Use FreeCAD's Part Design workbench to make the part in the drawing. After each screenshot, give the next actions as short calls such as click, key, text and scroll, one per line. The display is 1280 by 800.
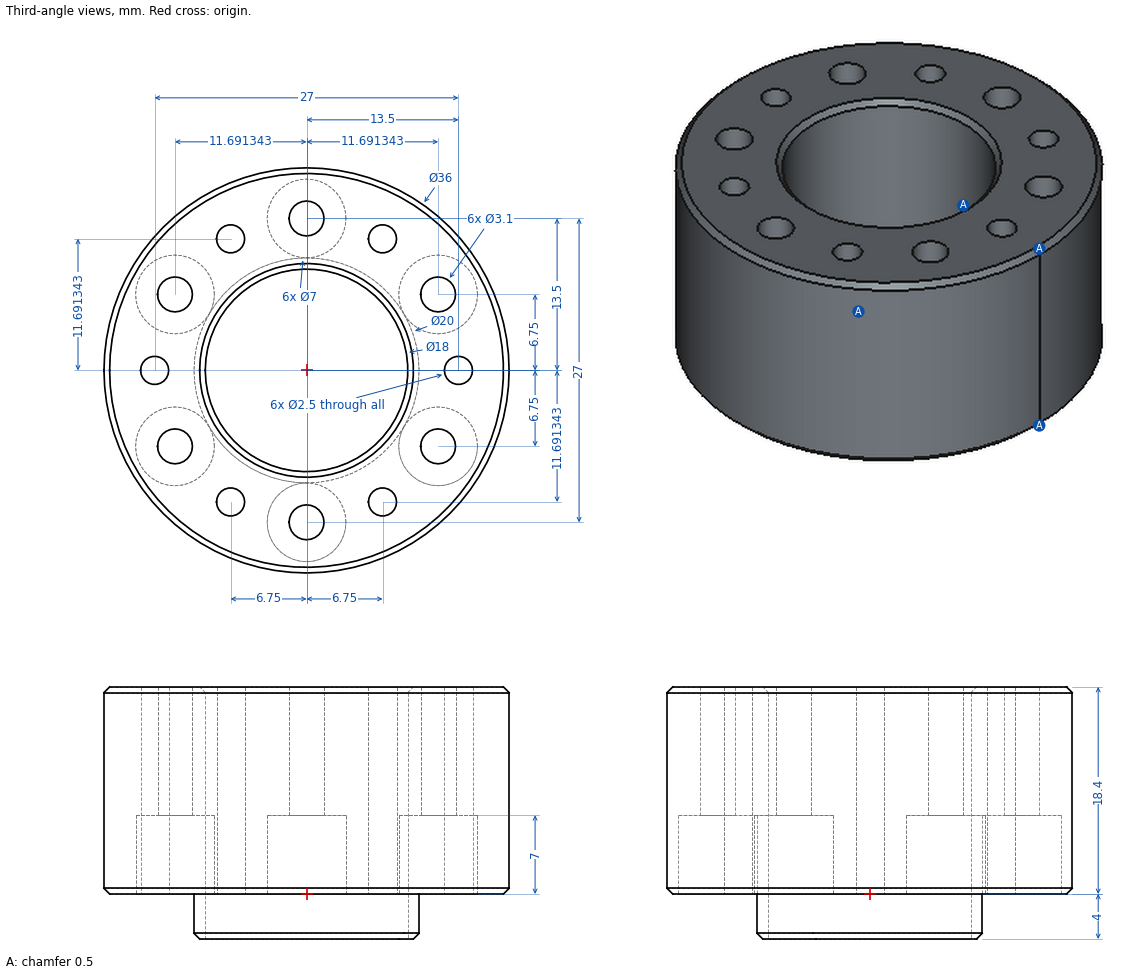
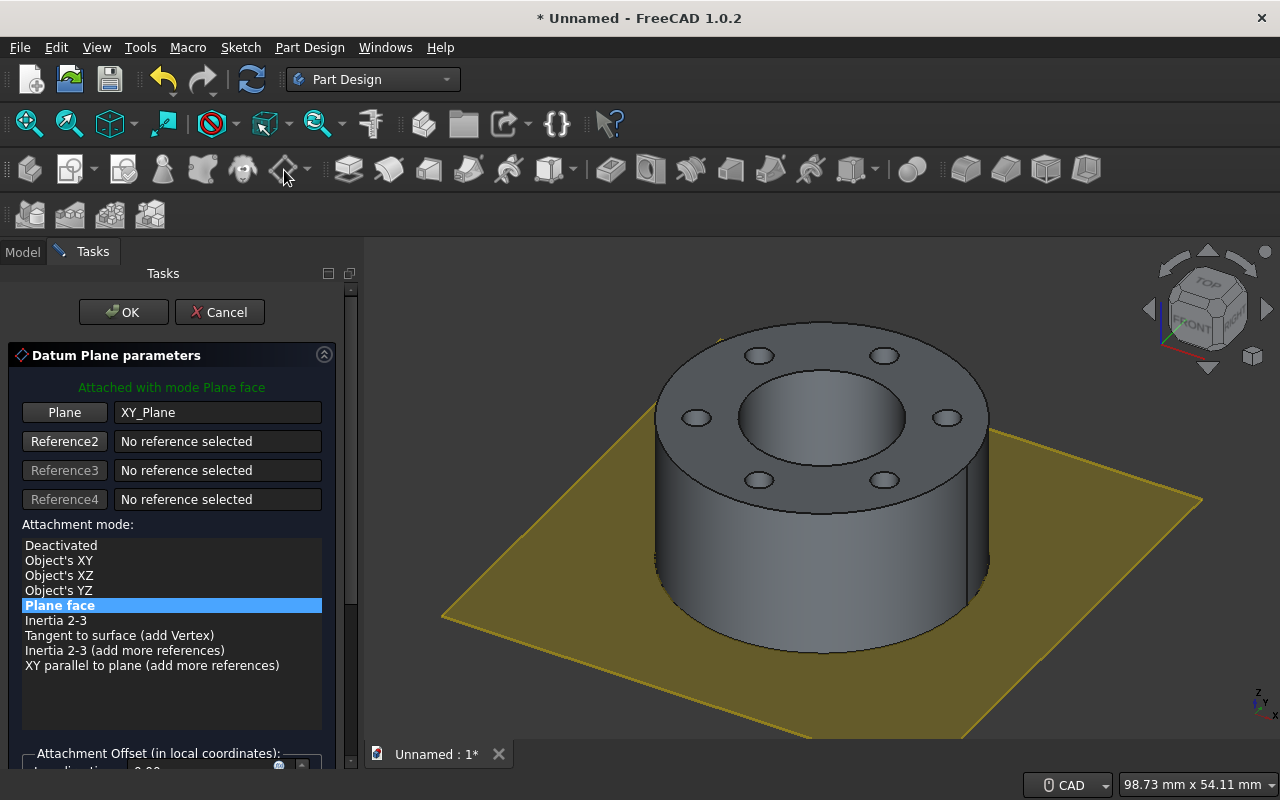
scroll(351, 526, down, 3)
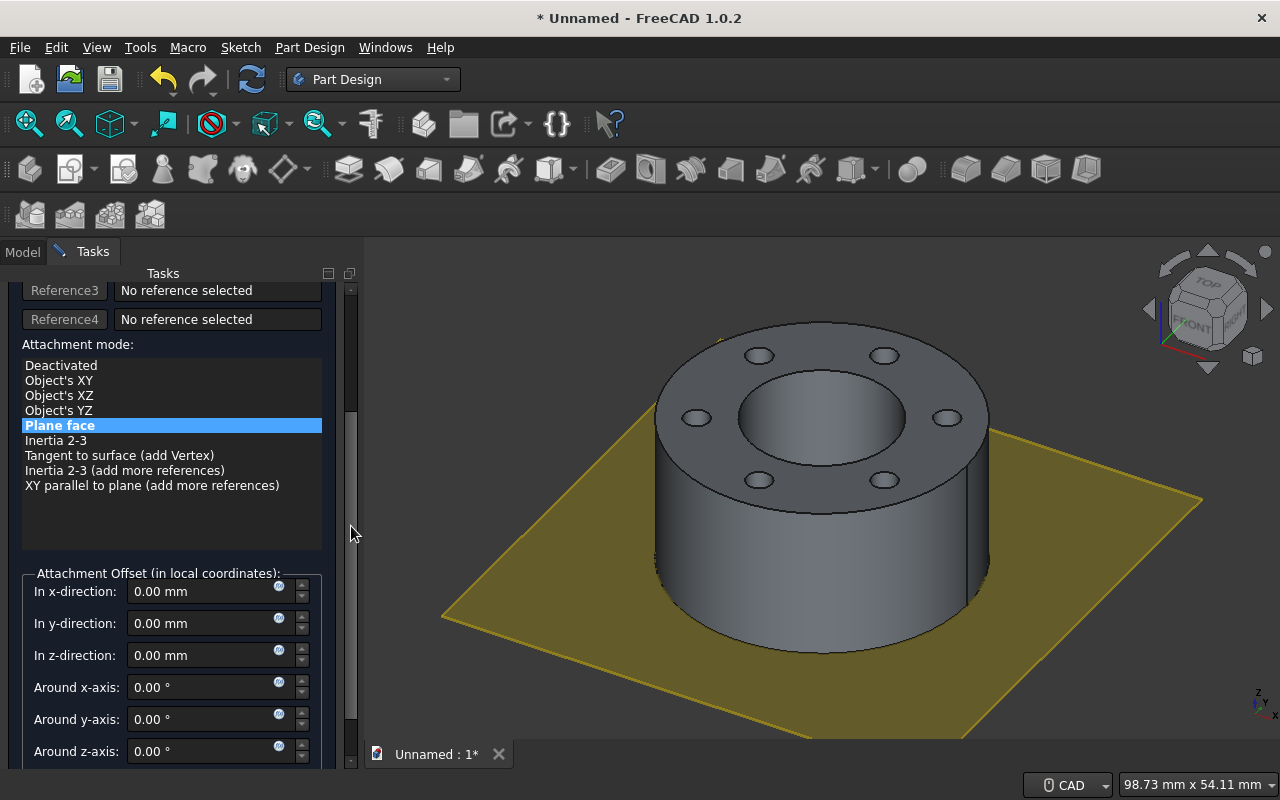
triple_click(210, 655)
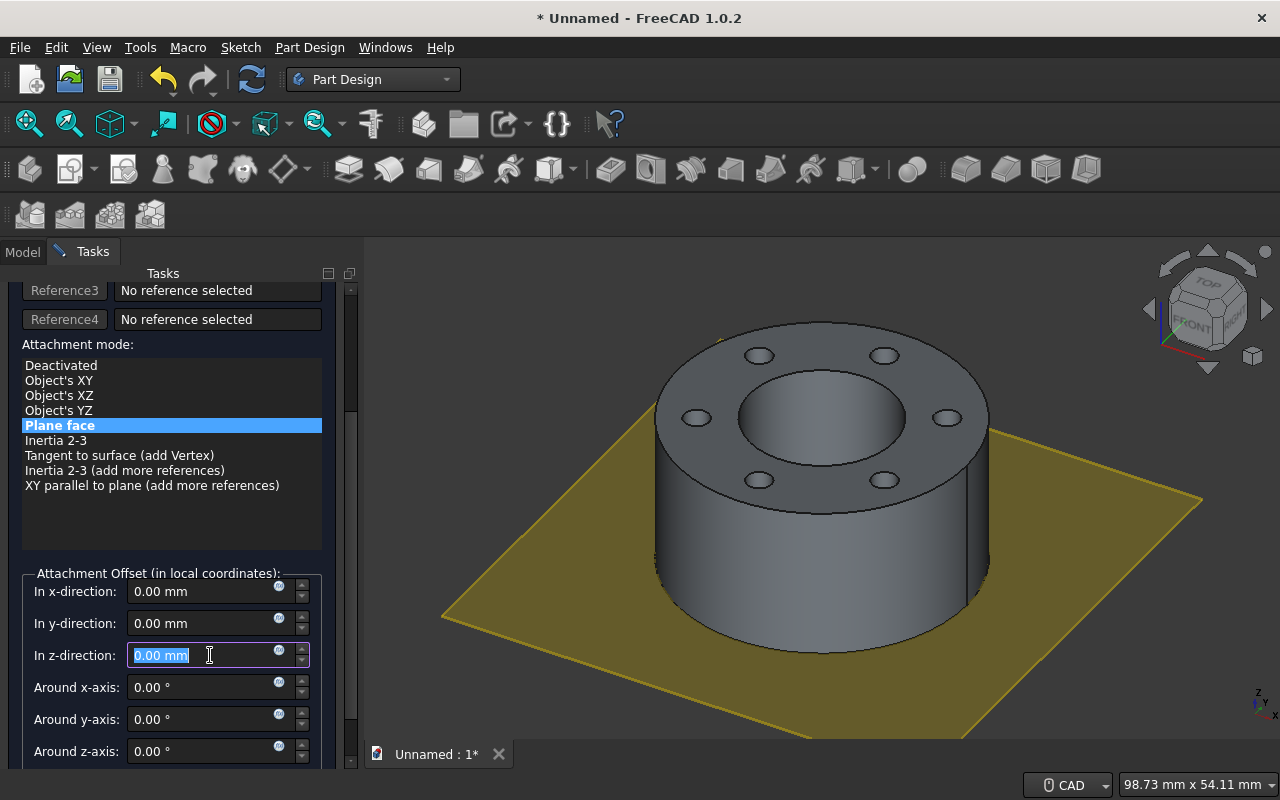
text(-4)
key(Tab)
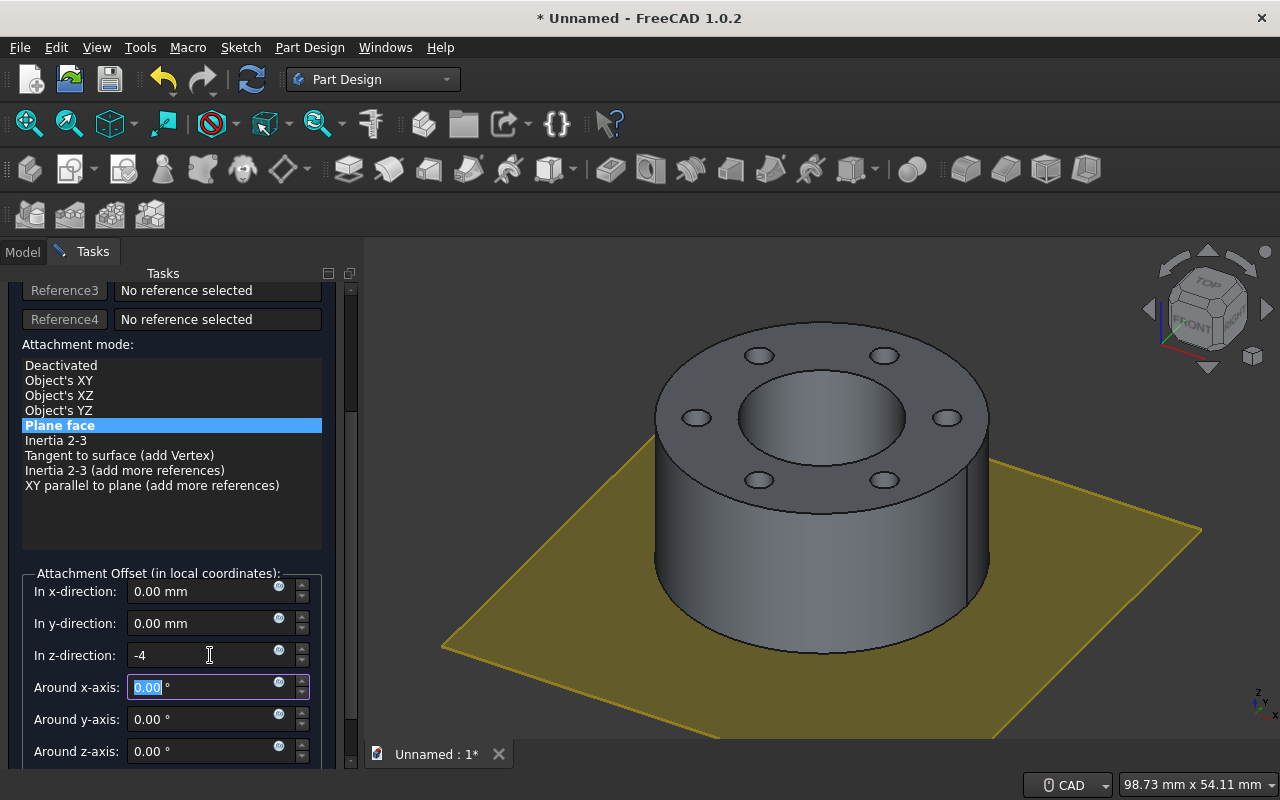
scroll(351, 526, up, 4)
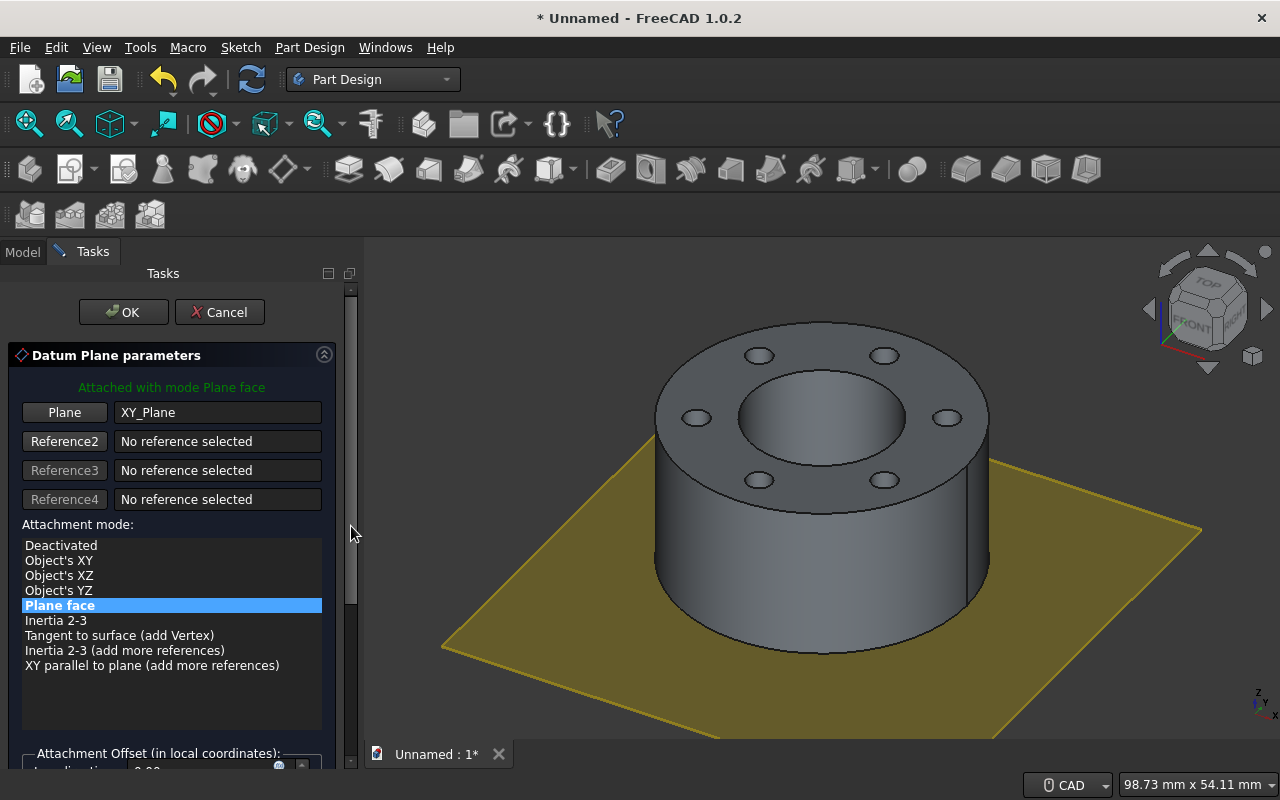
click(124, 312)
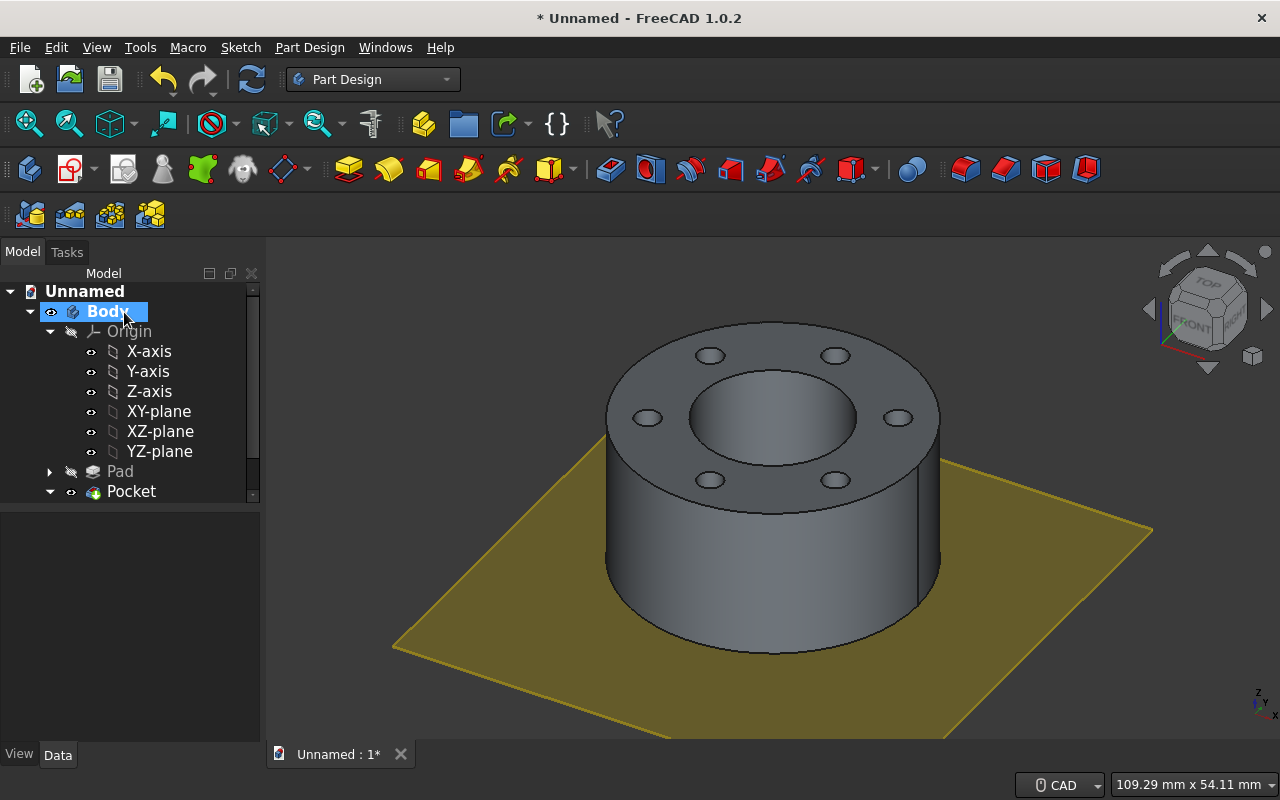
scroll(100, 387, down, 3)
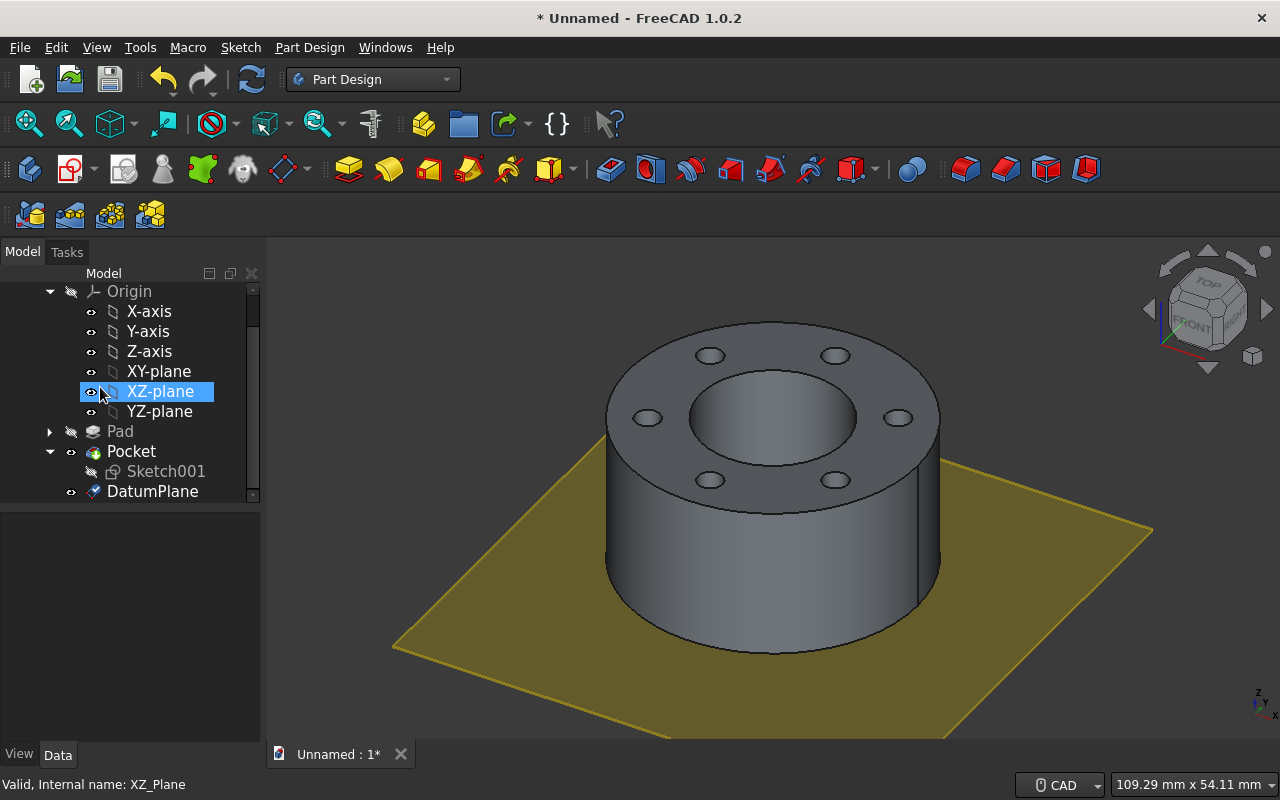
click(116, 492)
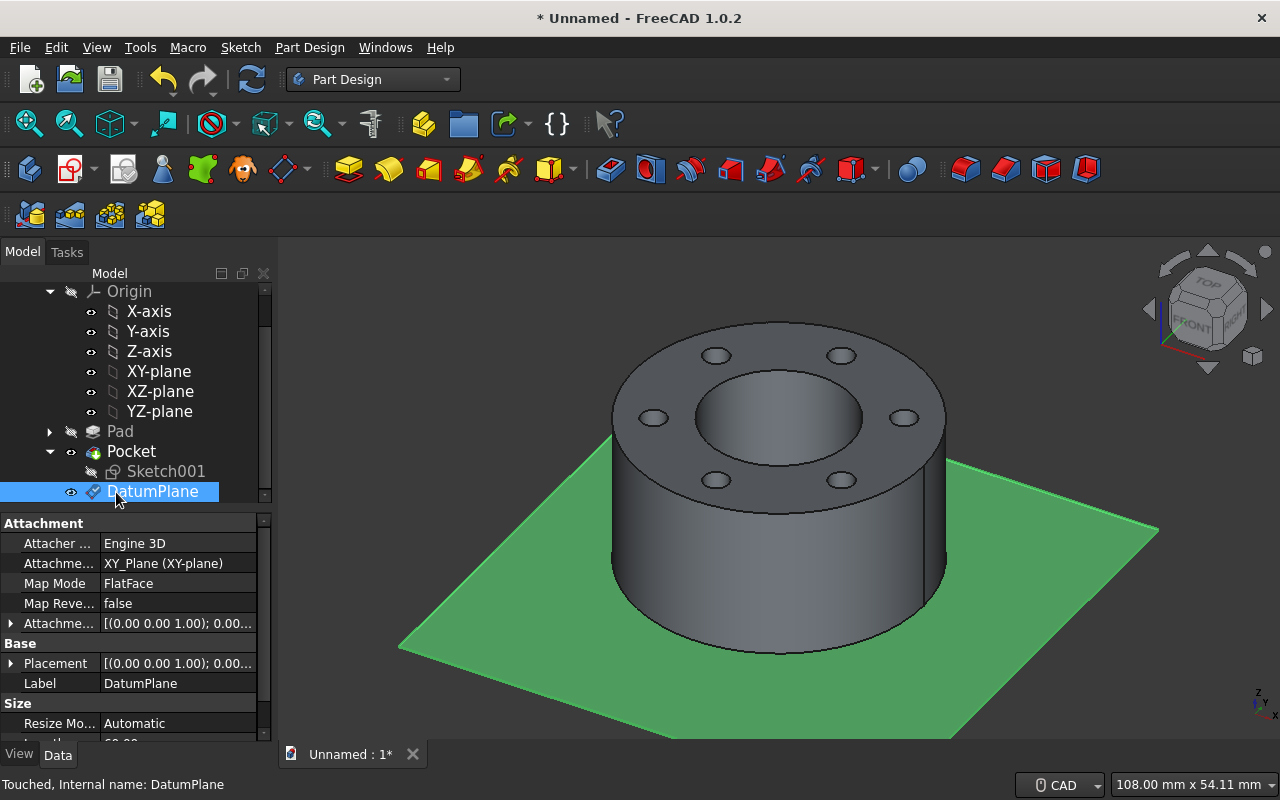
click(70, 170)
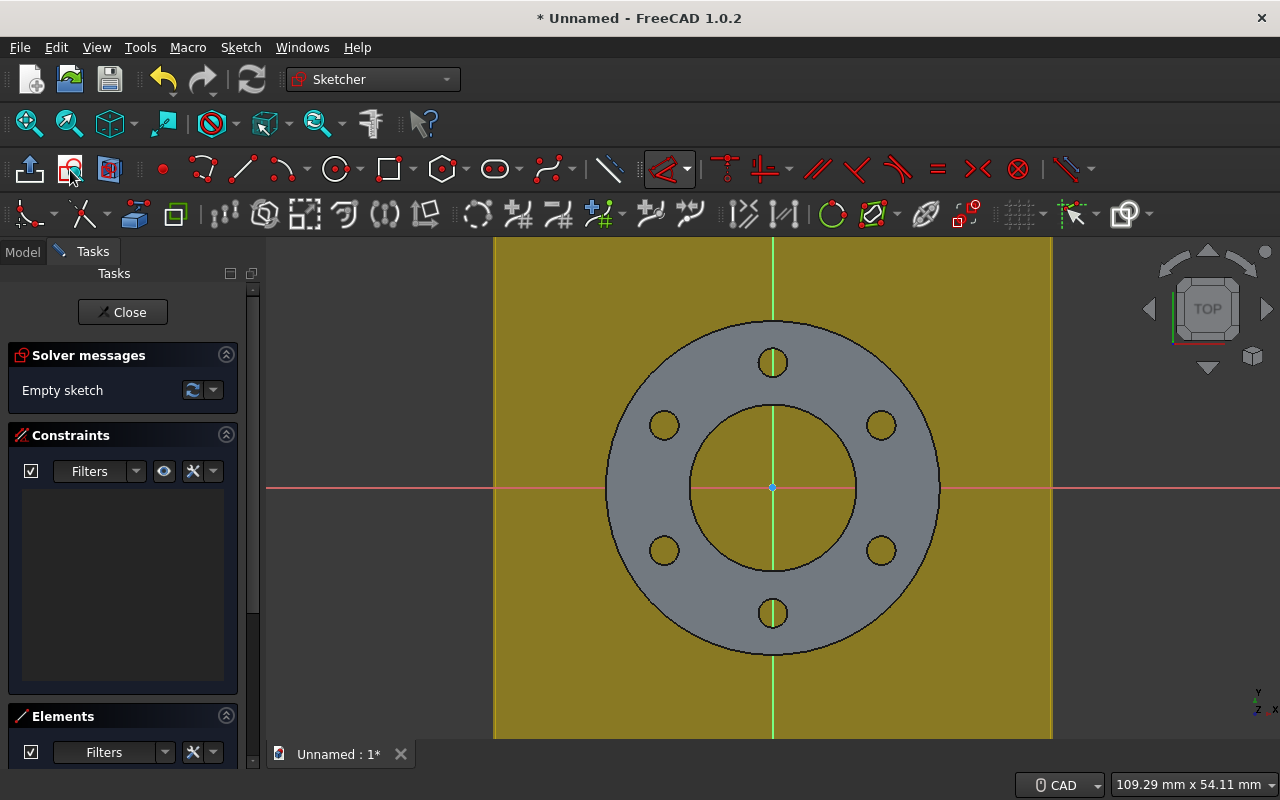
key(q)
key(s)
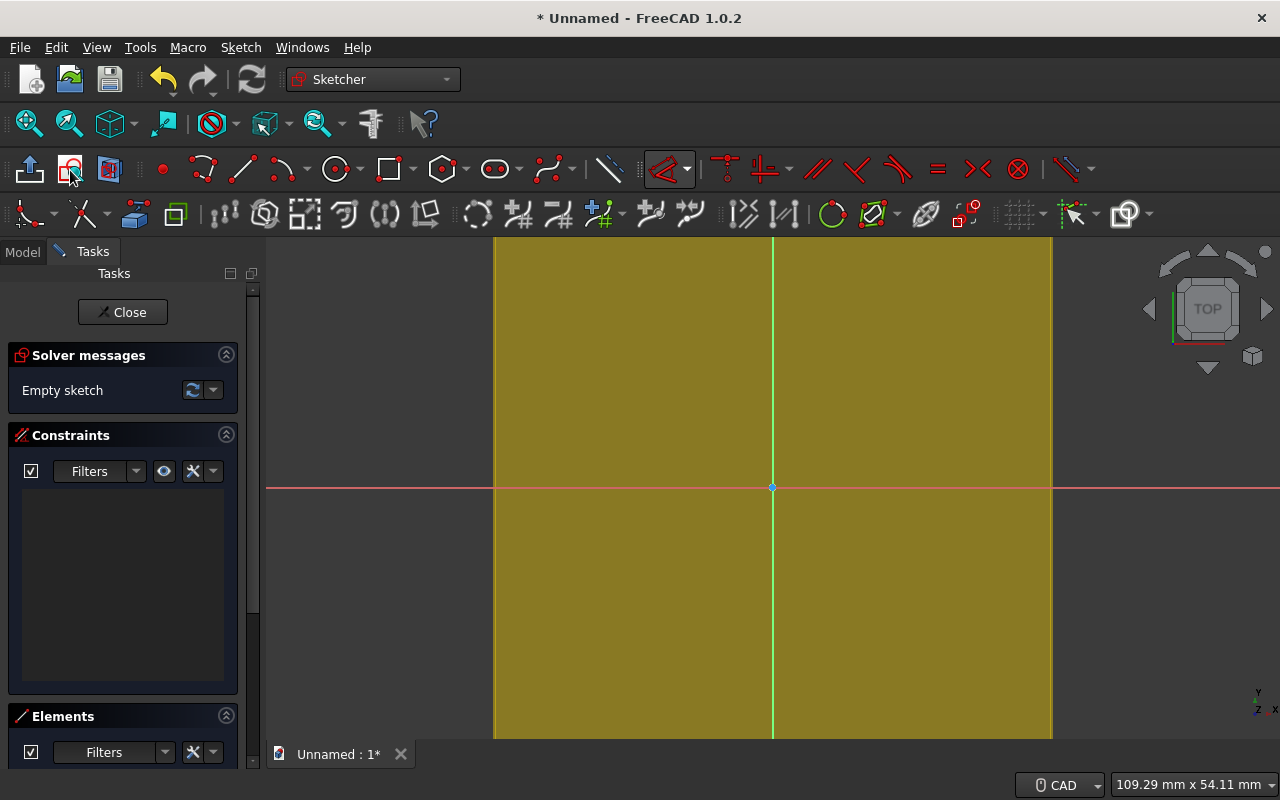
scroll(856, 488, up, 3)